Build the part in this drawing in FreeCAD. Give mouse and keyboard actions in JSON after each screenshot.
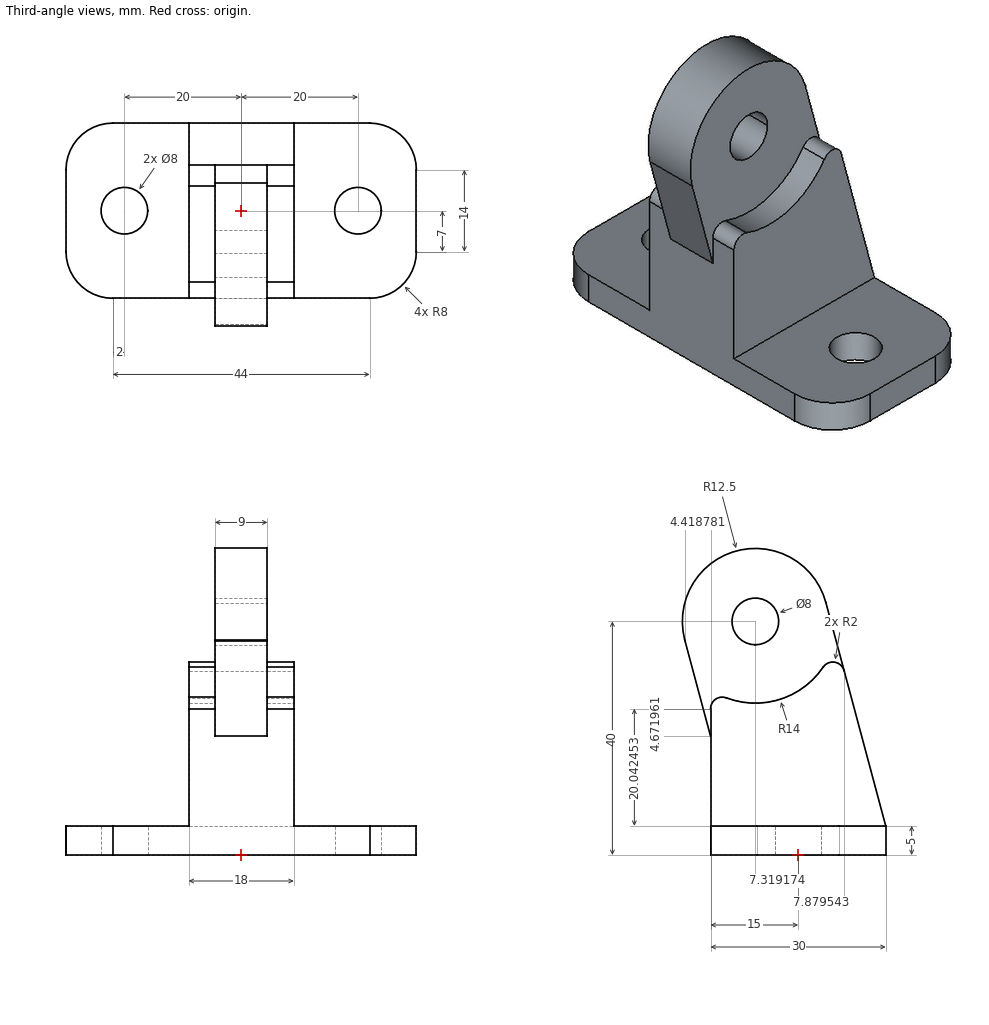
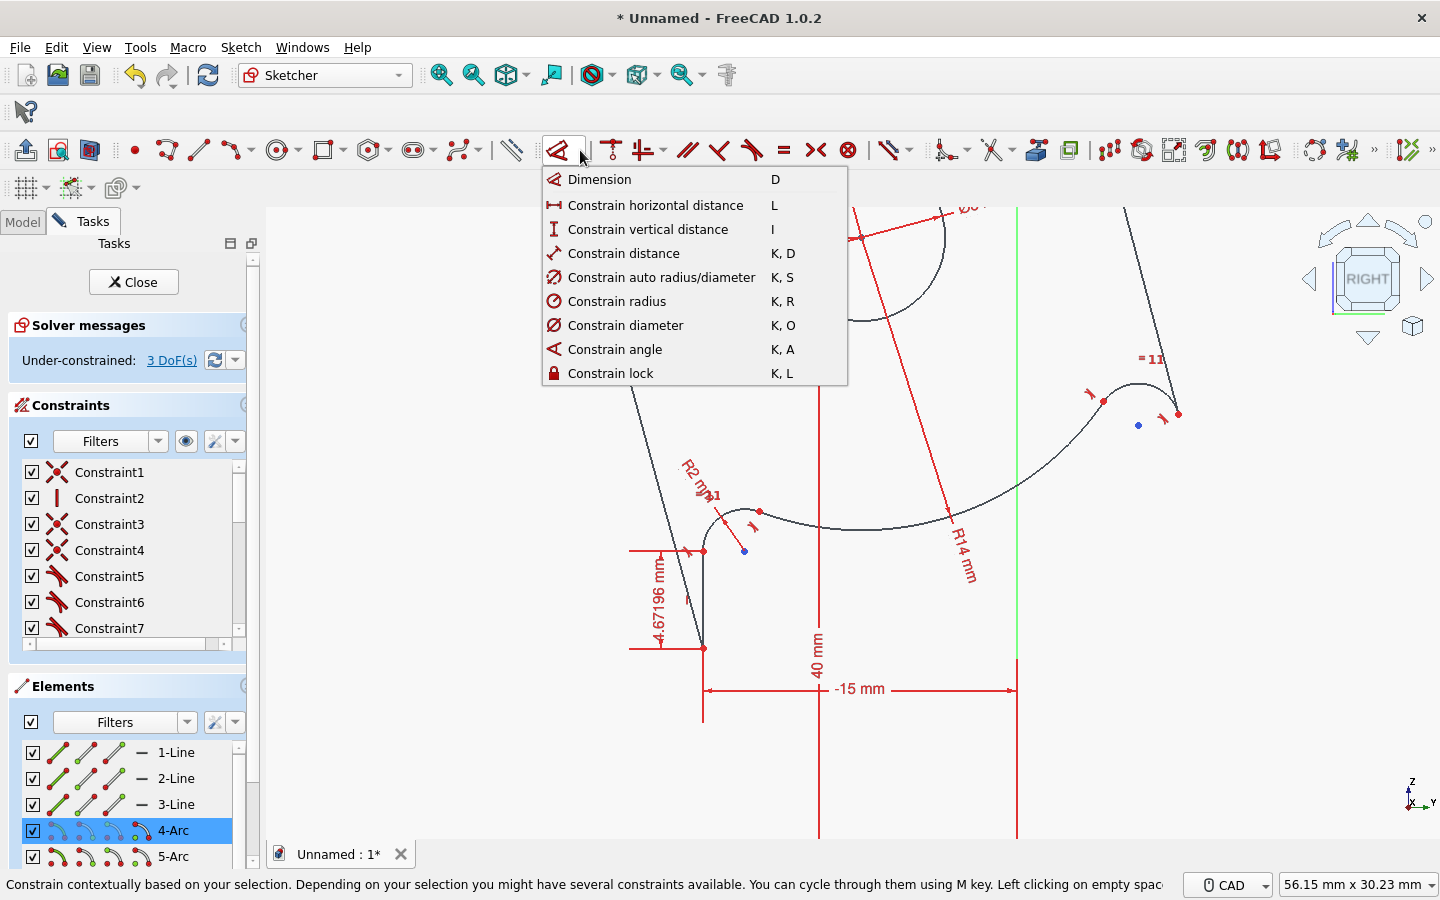
{"action": "left_click", "coordinate": [695, 205]}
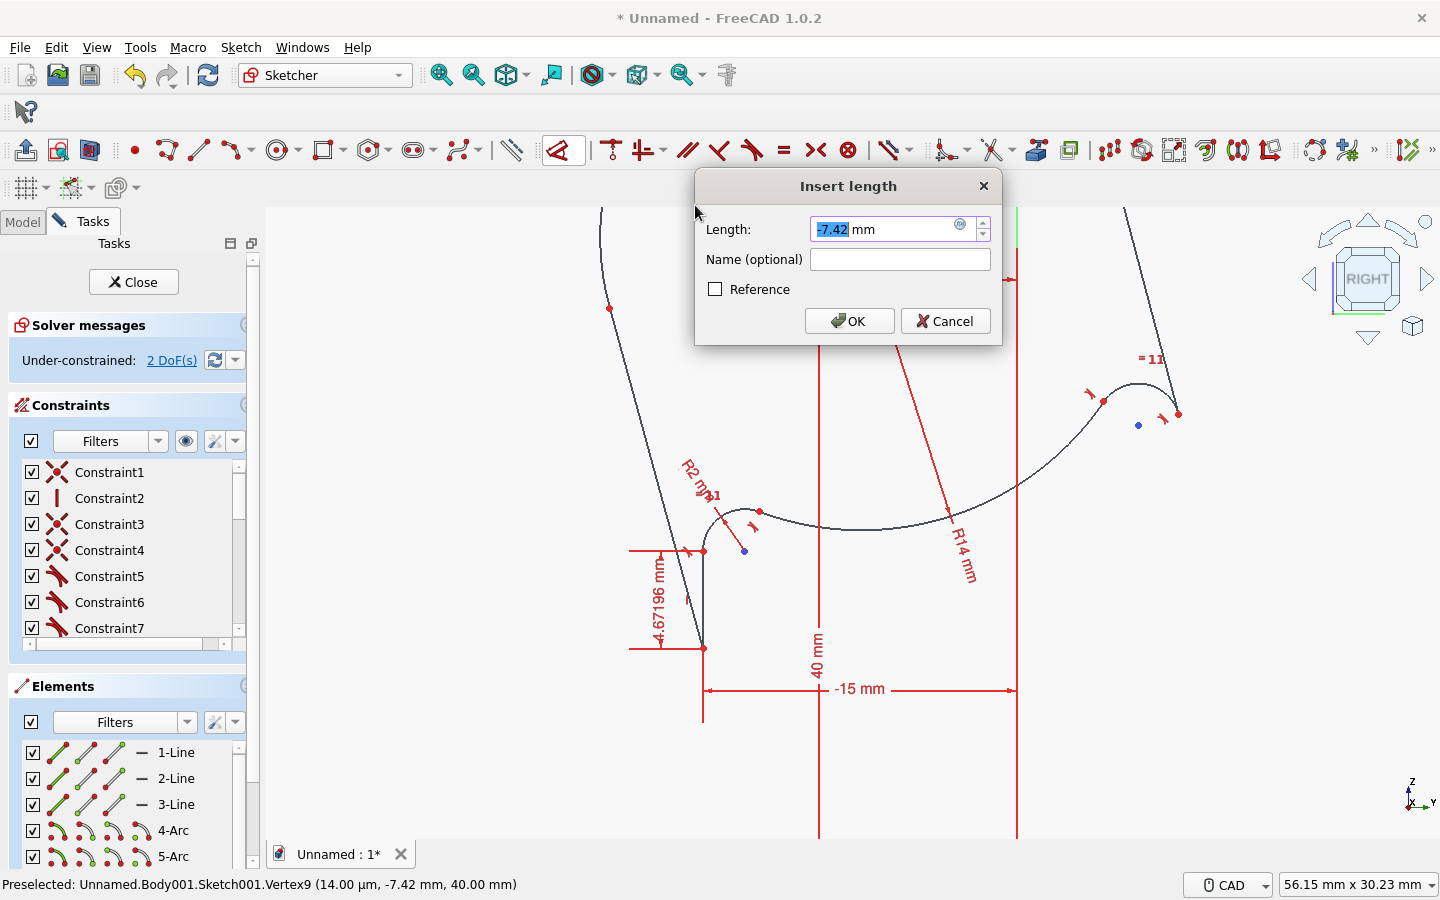
{"action": "type", "text": "-7.319174"}
{"action": "key", "text": "Return"}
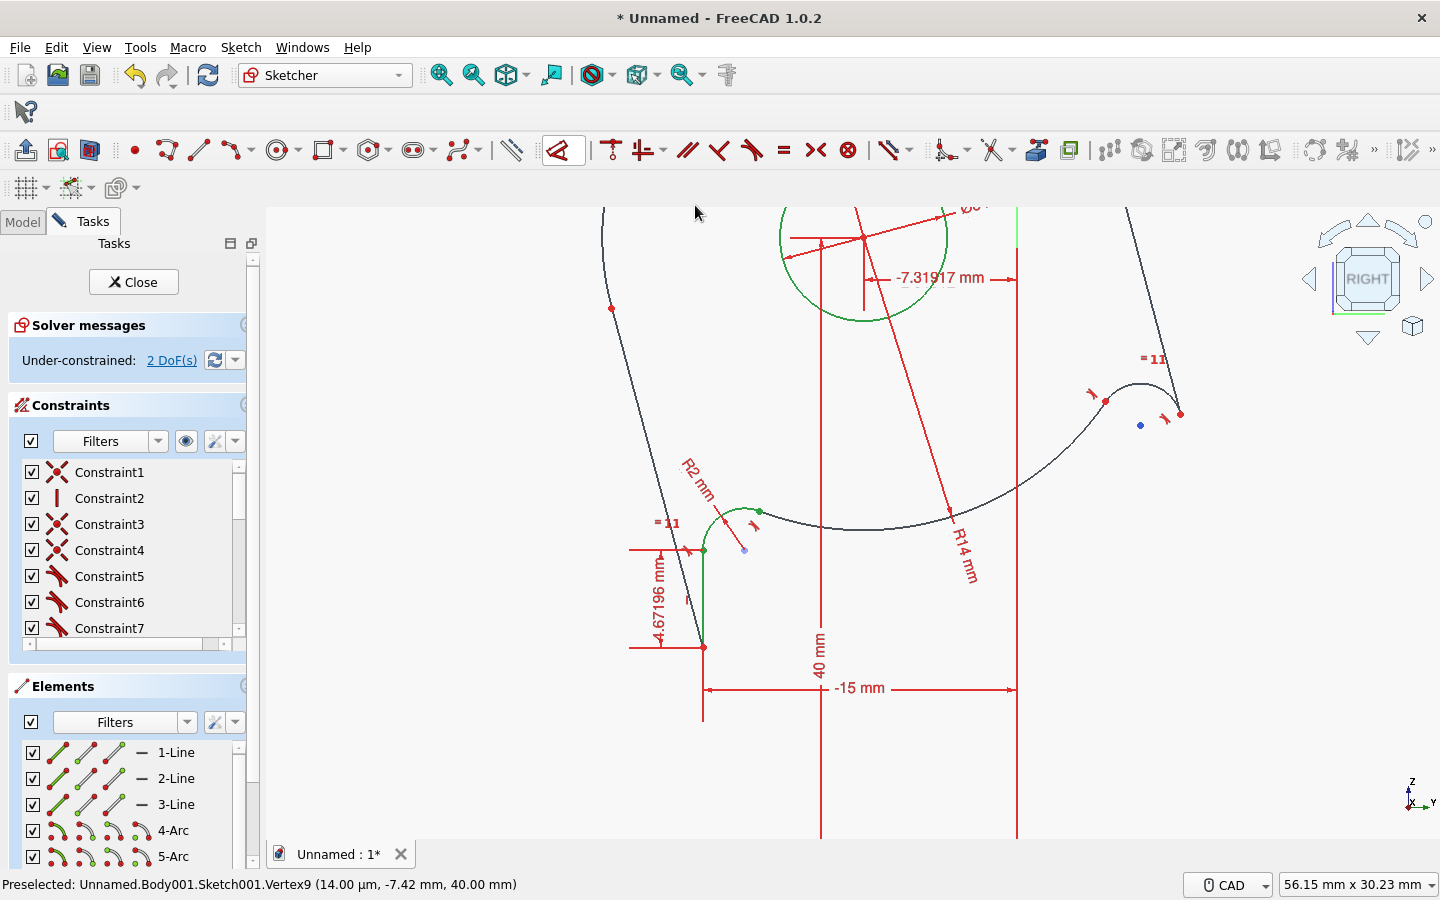
{"action": "left_click", "coordinate": [1181, 415]}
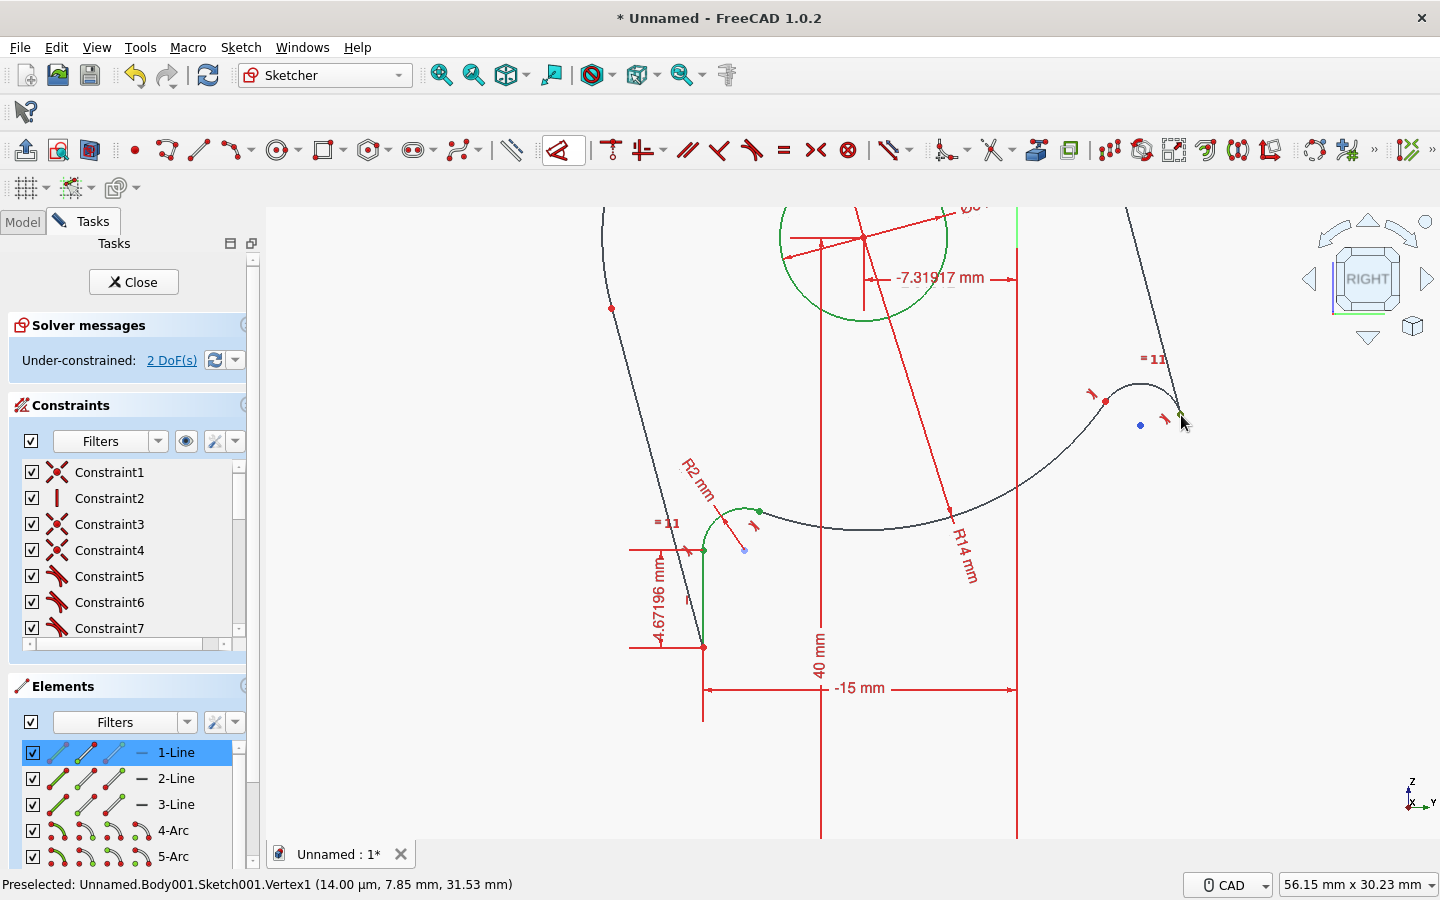
{"action": "key", "text": "l"}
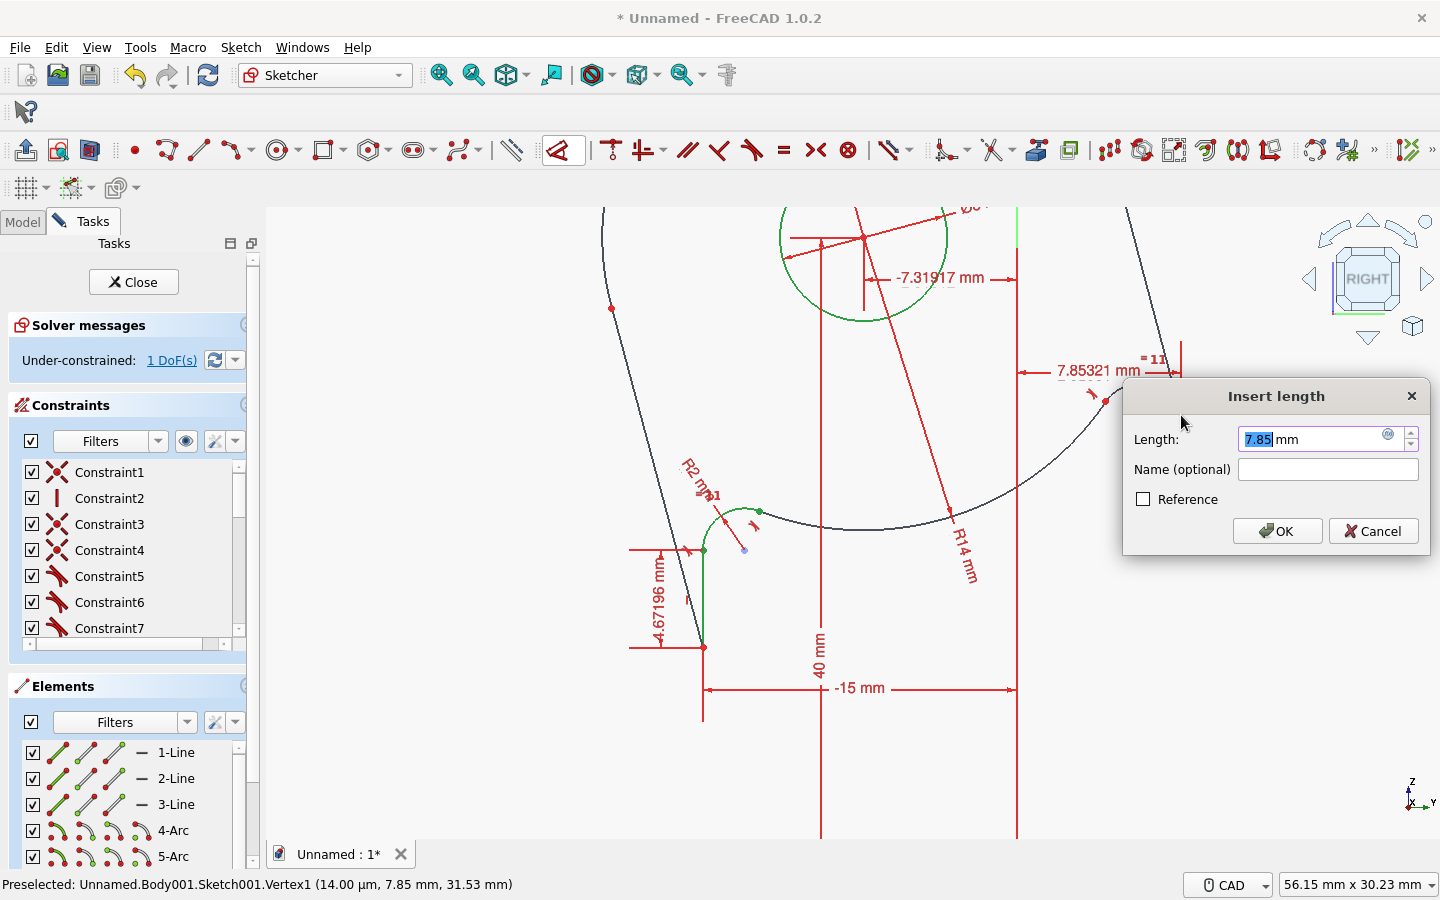
{"action": "type", "text": "7.879543"}
{"action": "key", "text": "Return"}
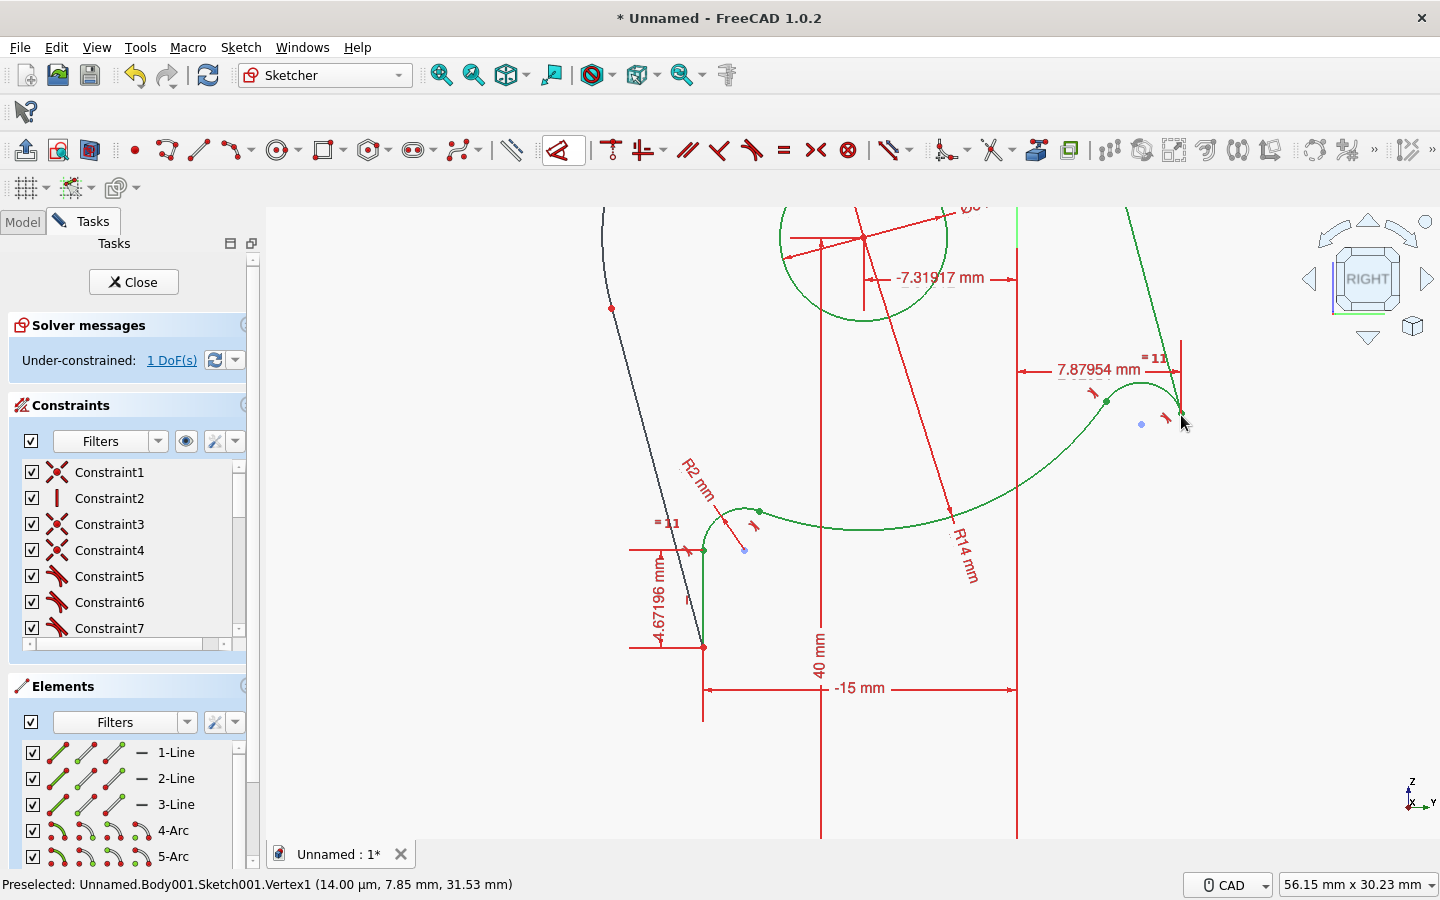
{"action": "left_click", "coordinate": [639, 410]}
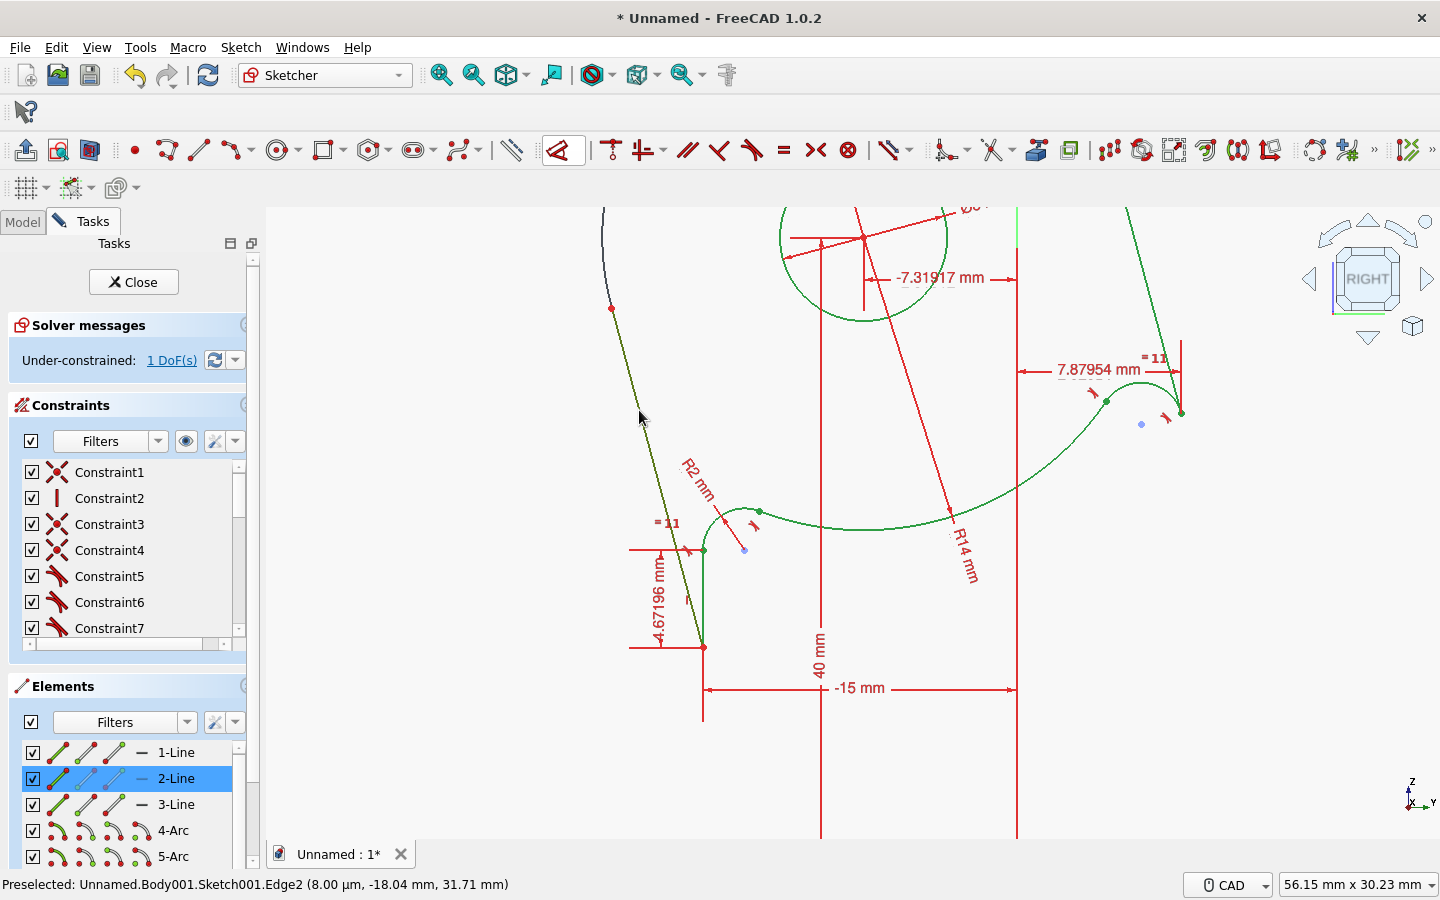
{"action": "key", "text": "l"}